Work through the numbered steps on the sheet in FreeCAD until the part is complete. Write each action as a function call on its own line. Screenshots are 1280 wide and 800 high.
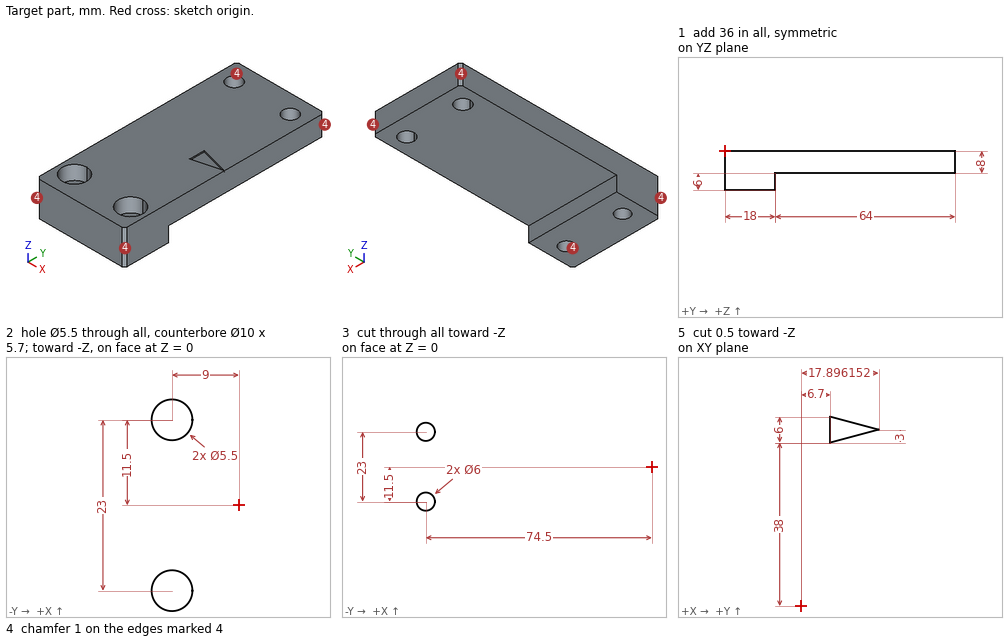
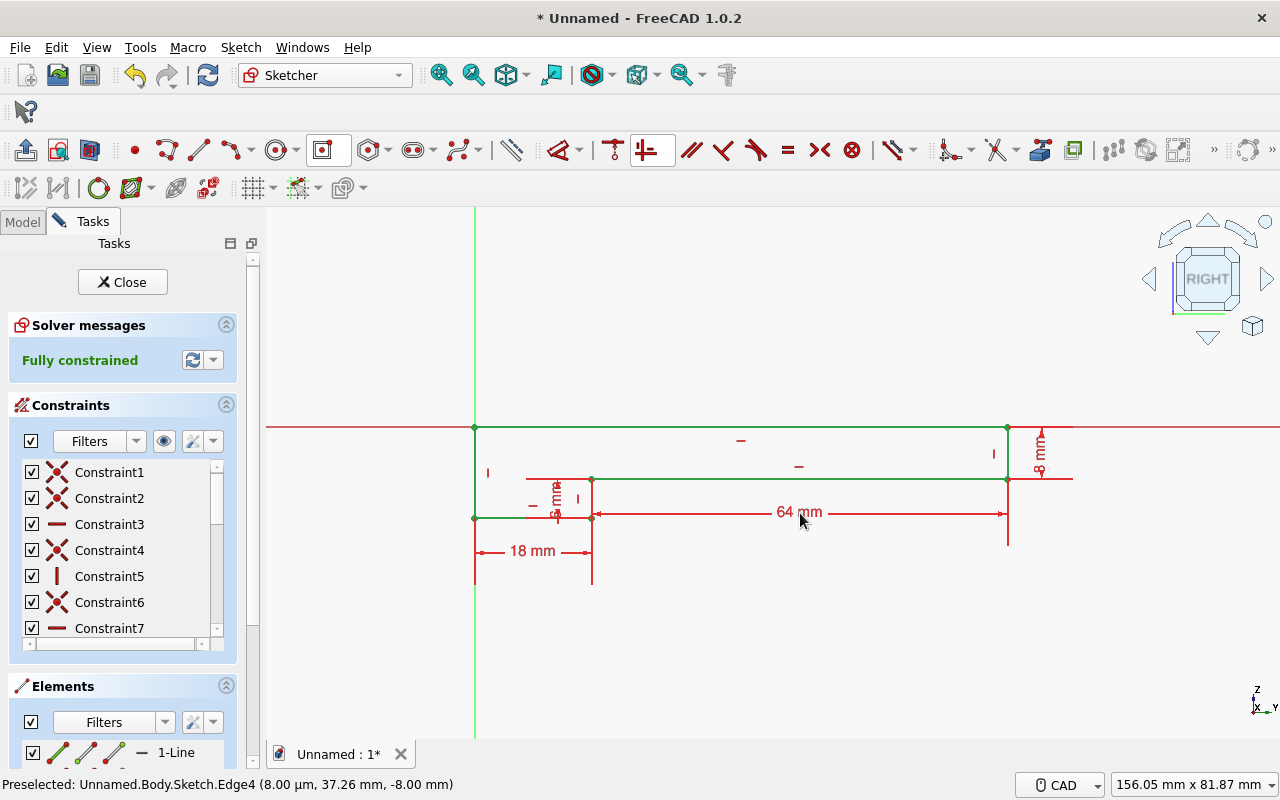
click(123, 282)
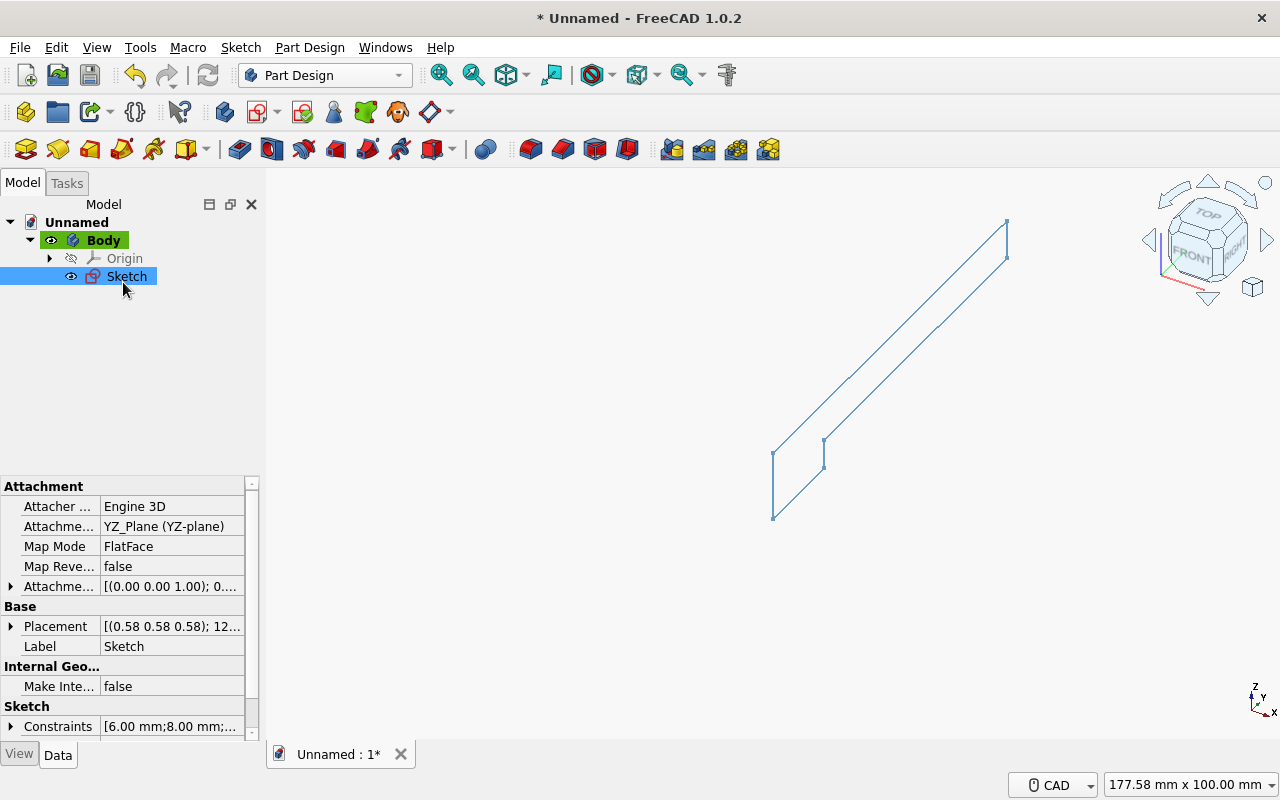
click(26, 150)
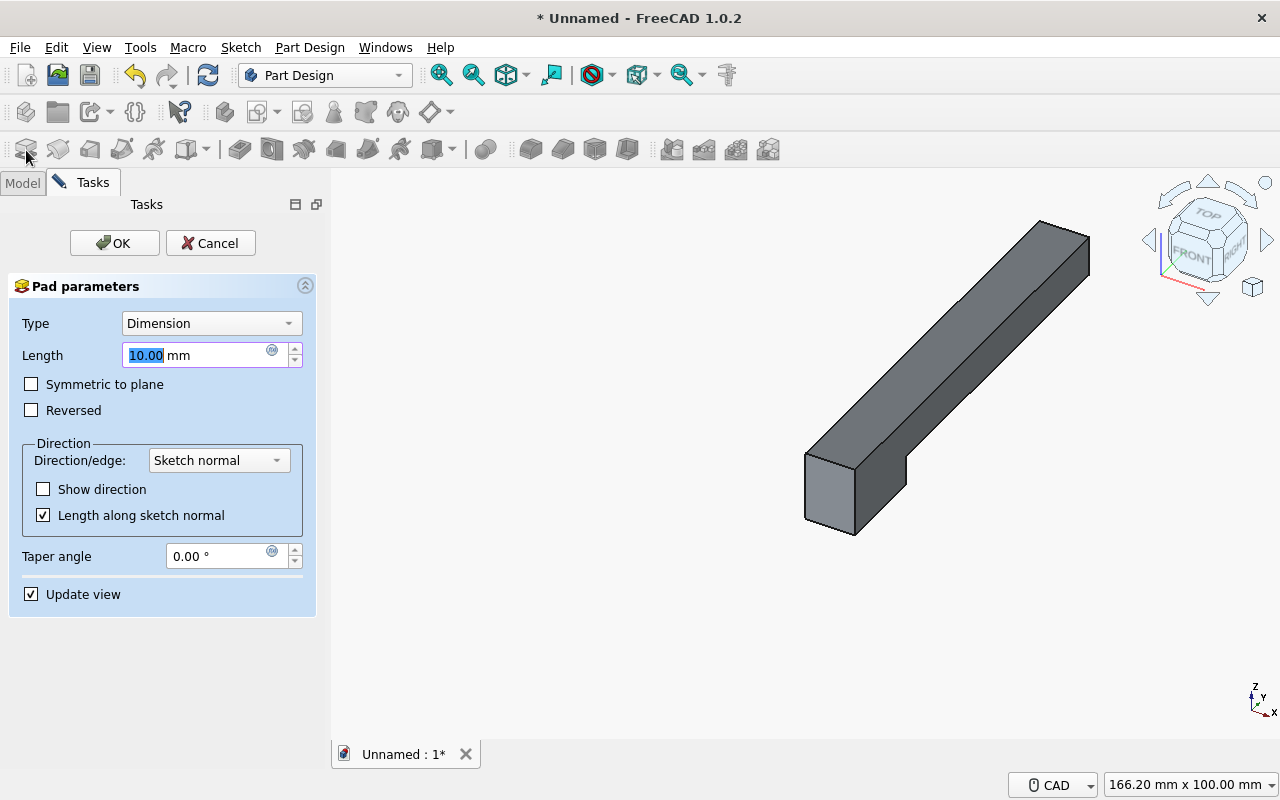
text(36)
key(Tab)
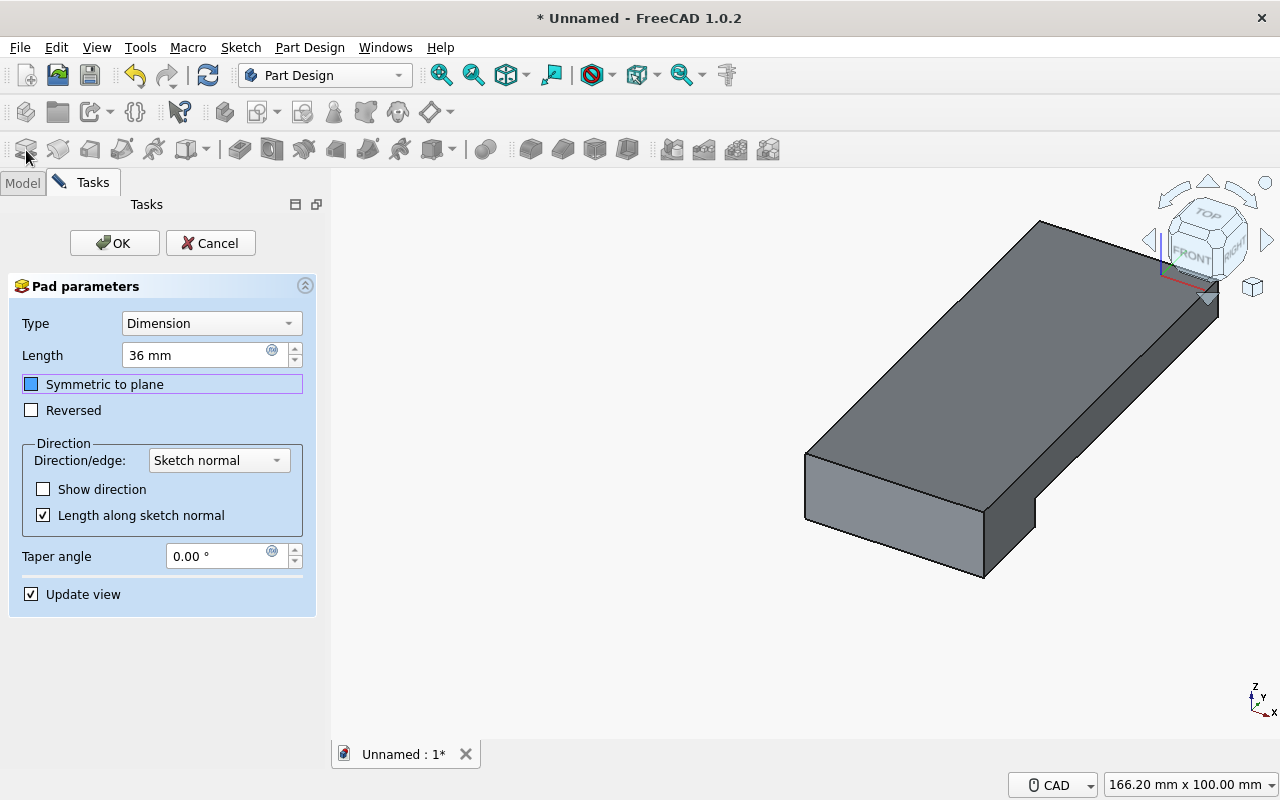
click(30, 384)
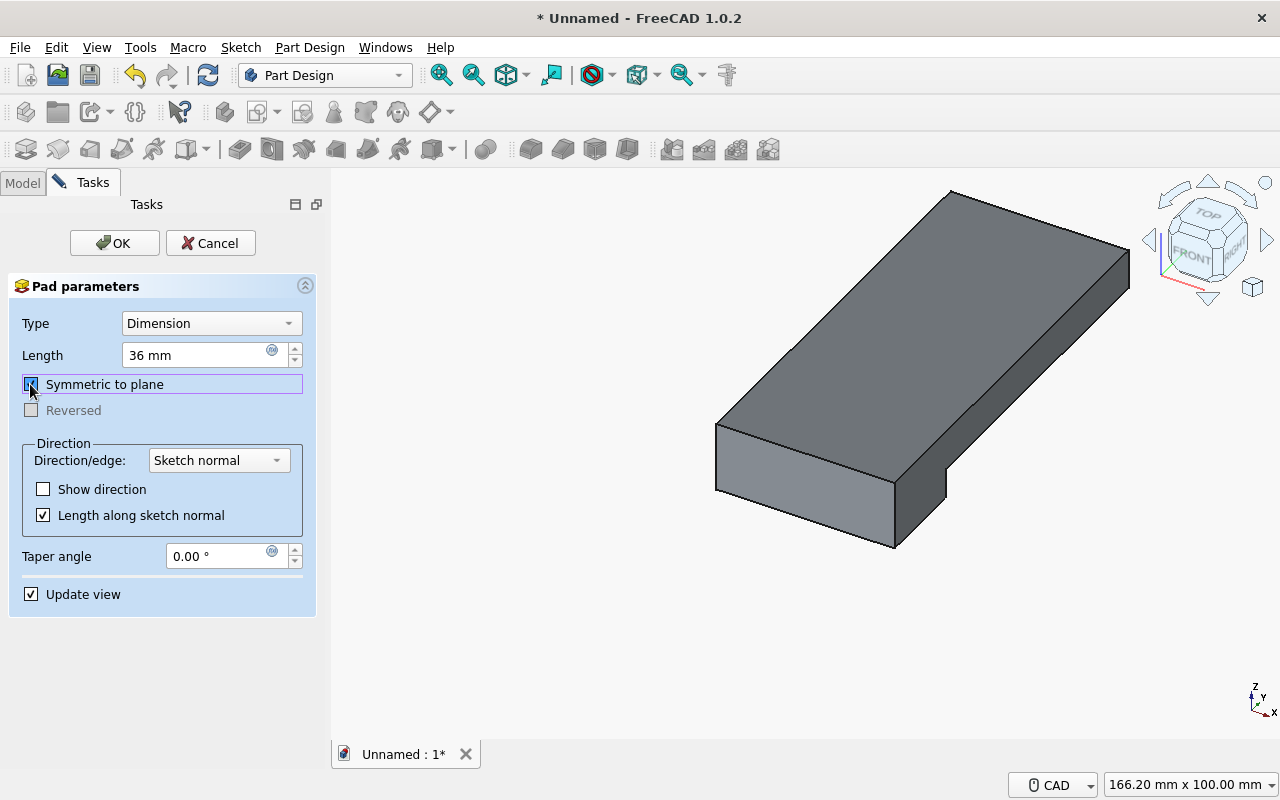
click(115, 243)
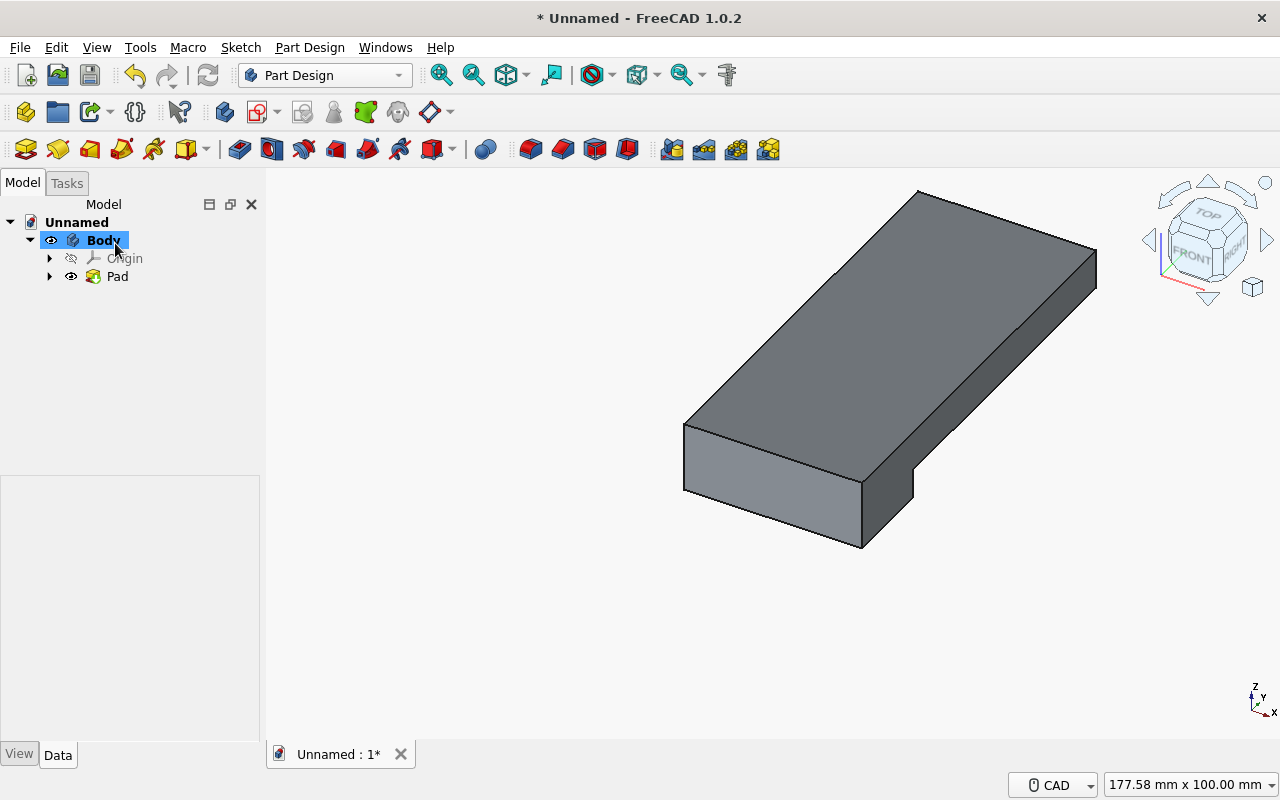
click(923, 303)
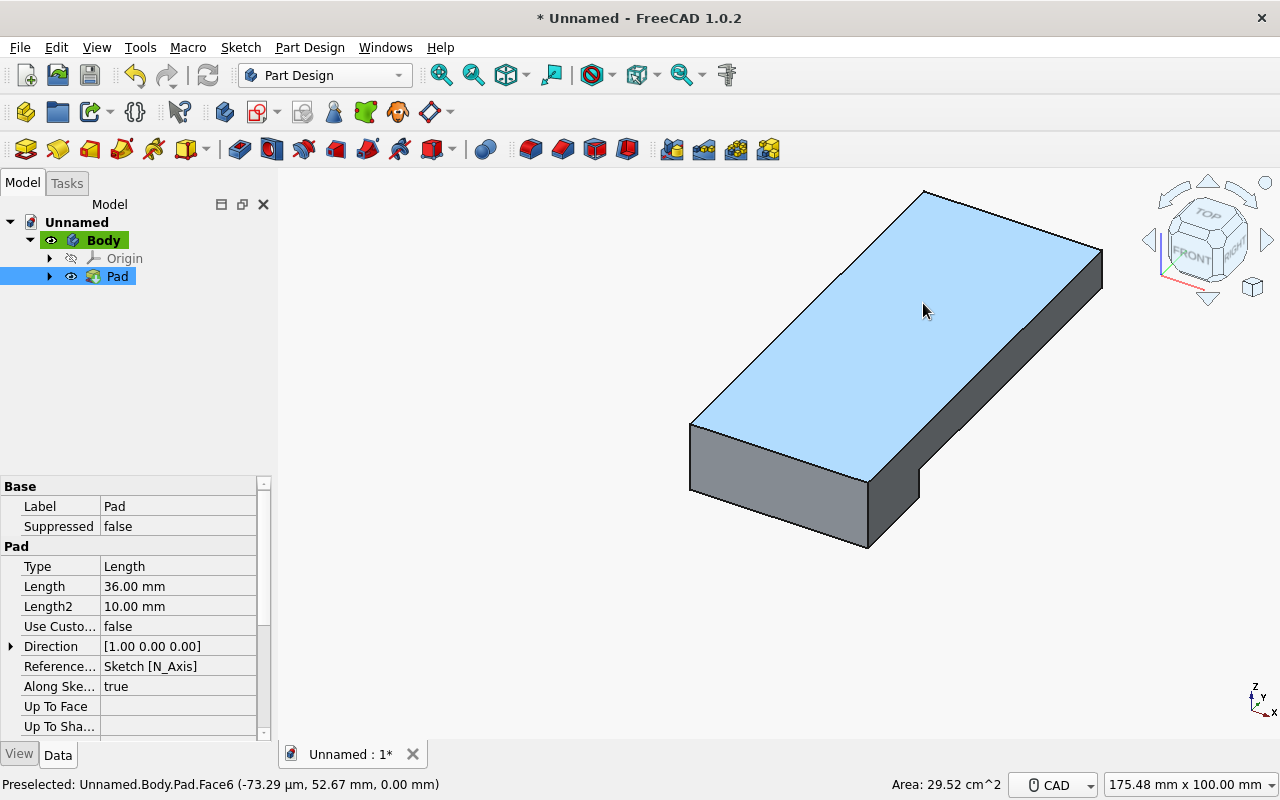
click(258, 112)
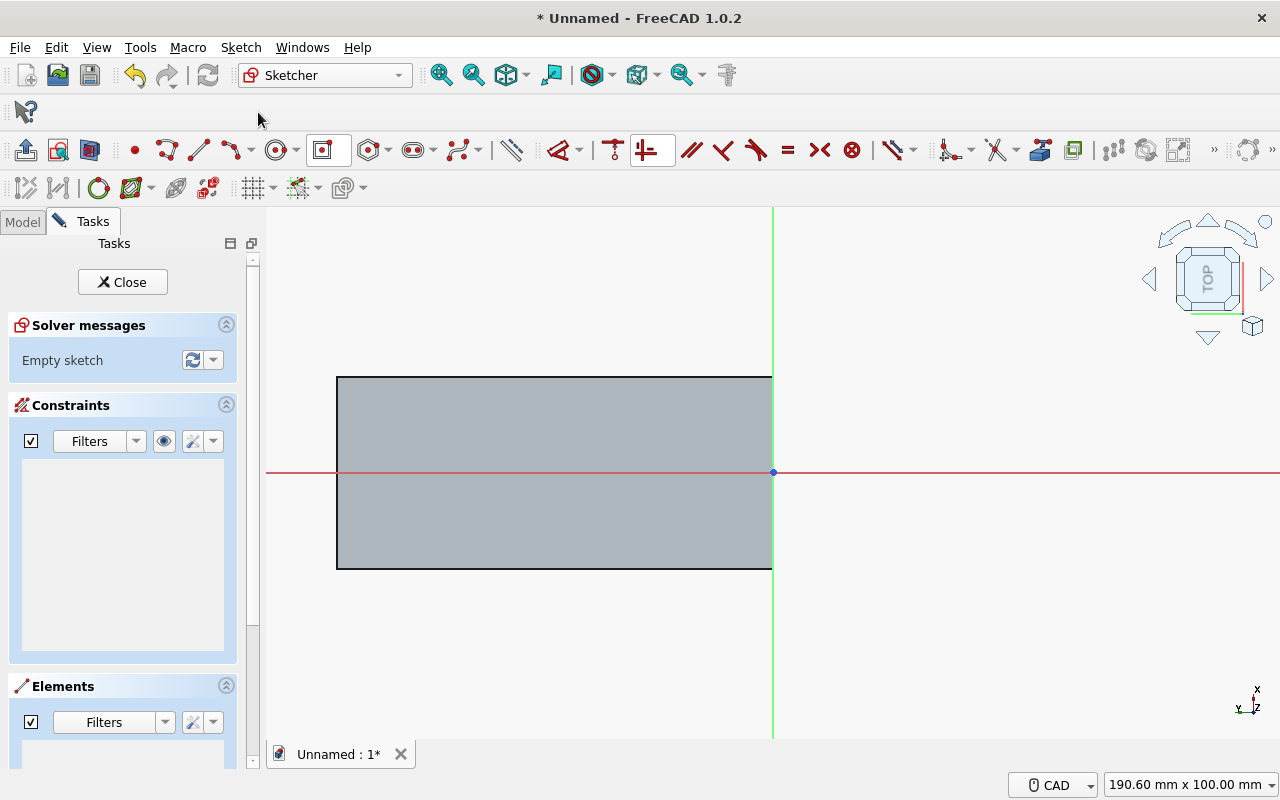
scroll(772, 473, up, 4)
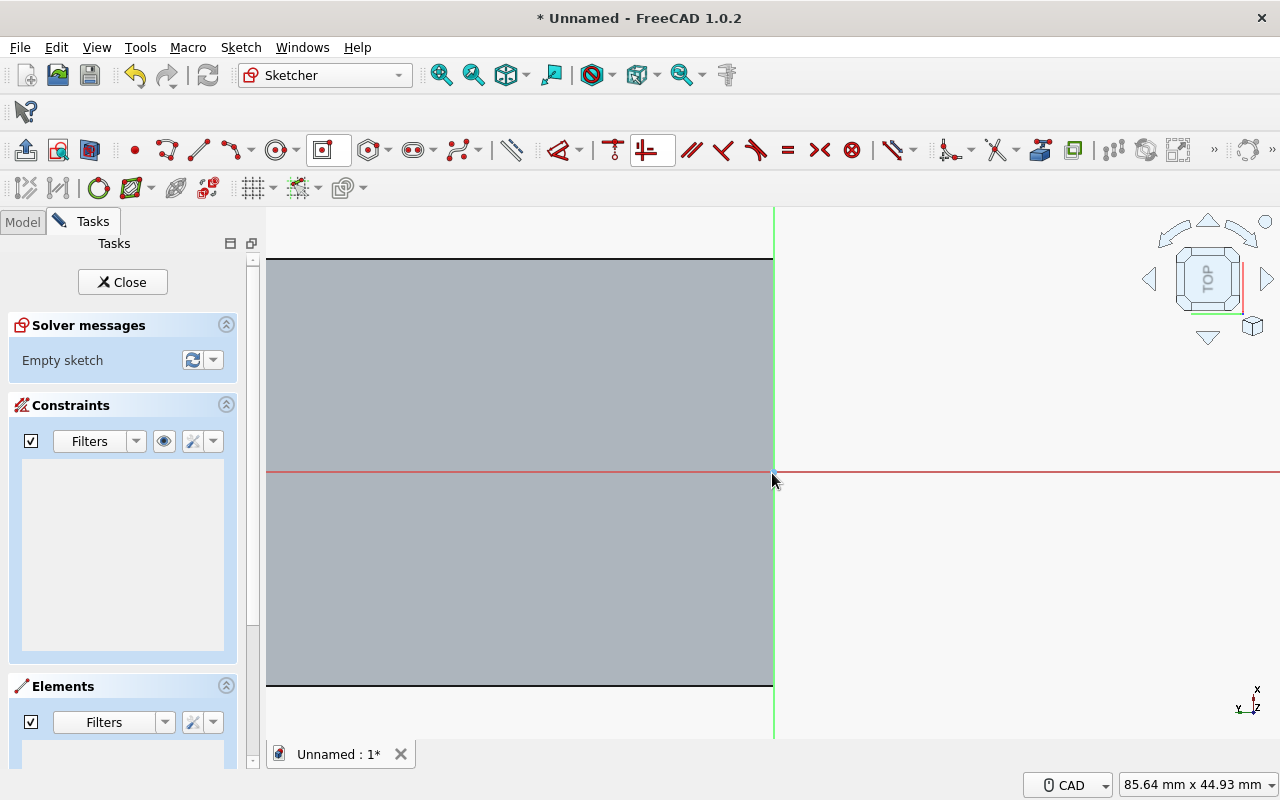
key(g)
key(c)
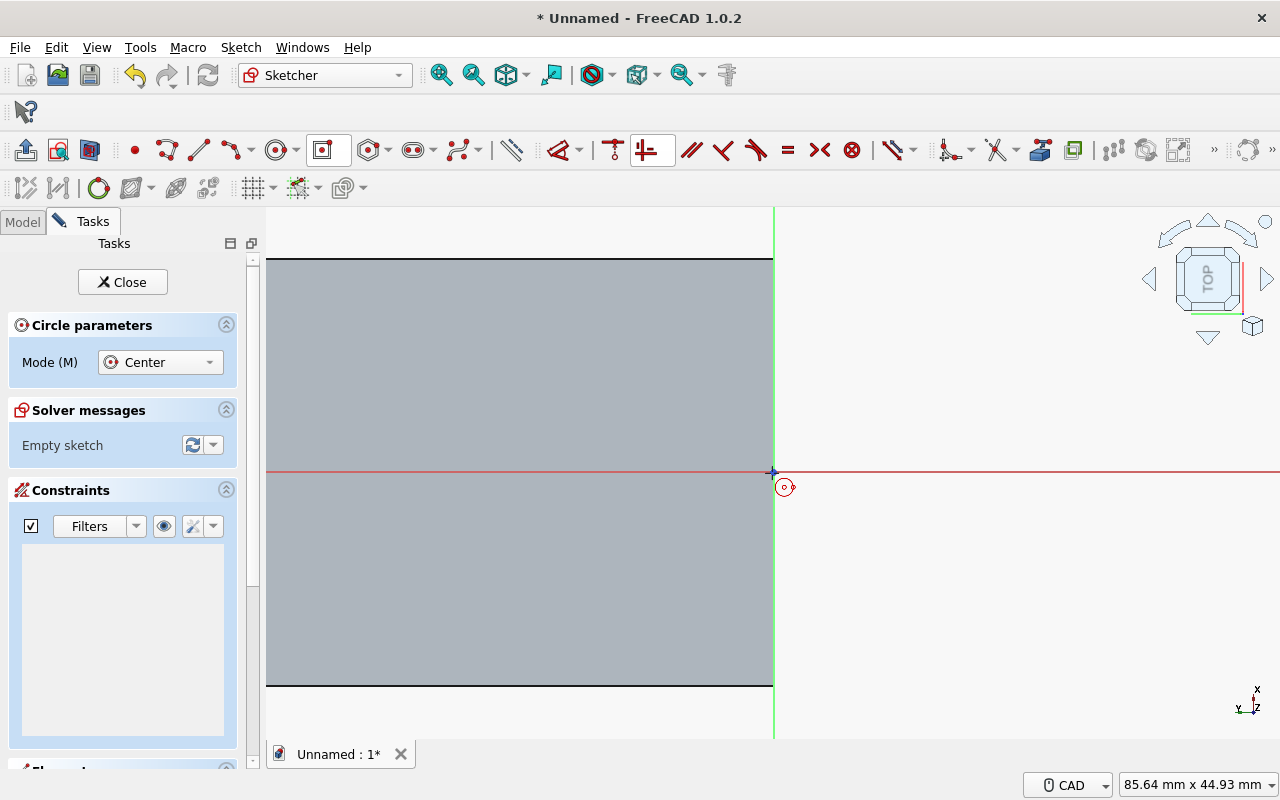
click(667, 336)
move(690, 313)